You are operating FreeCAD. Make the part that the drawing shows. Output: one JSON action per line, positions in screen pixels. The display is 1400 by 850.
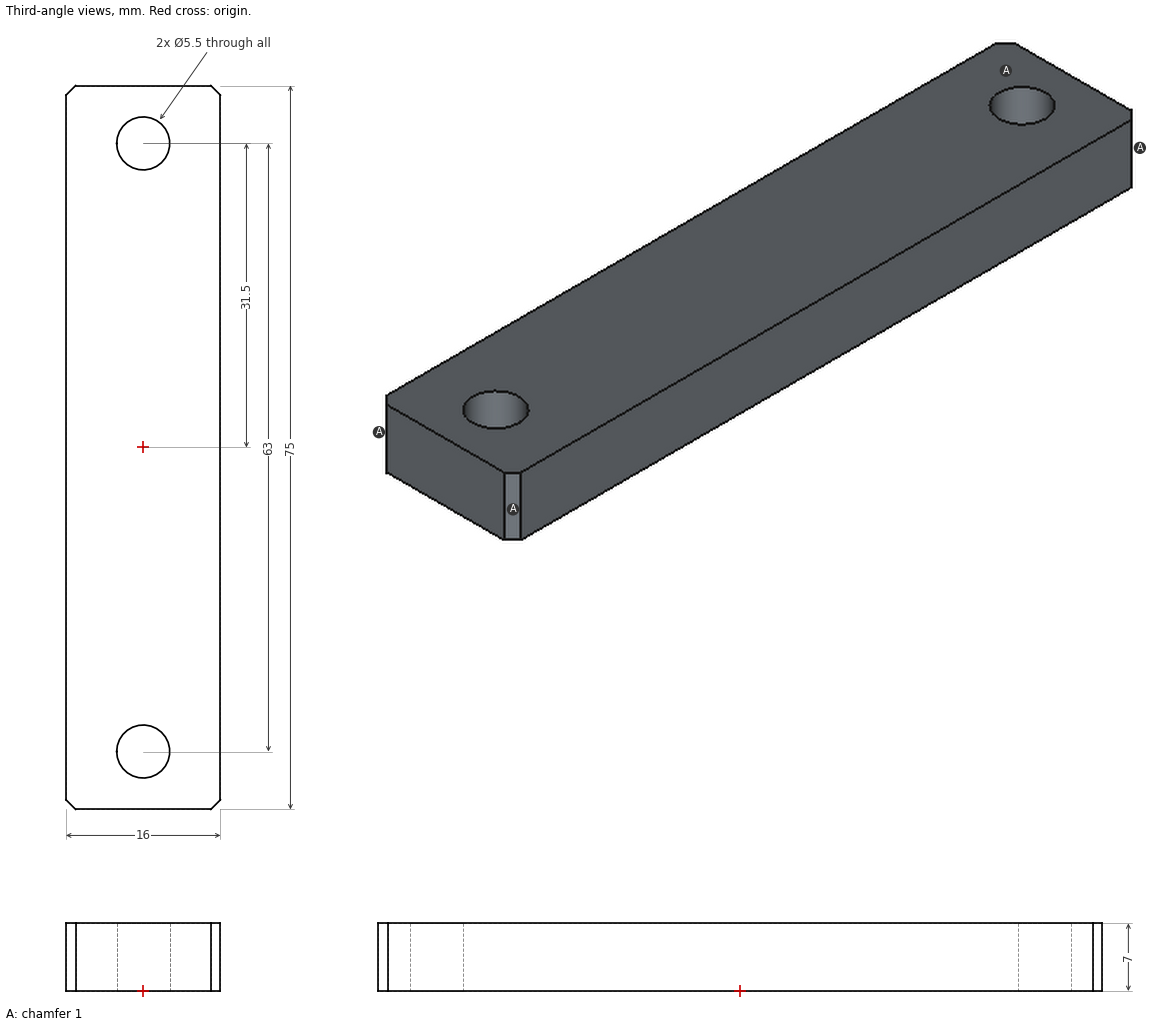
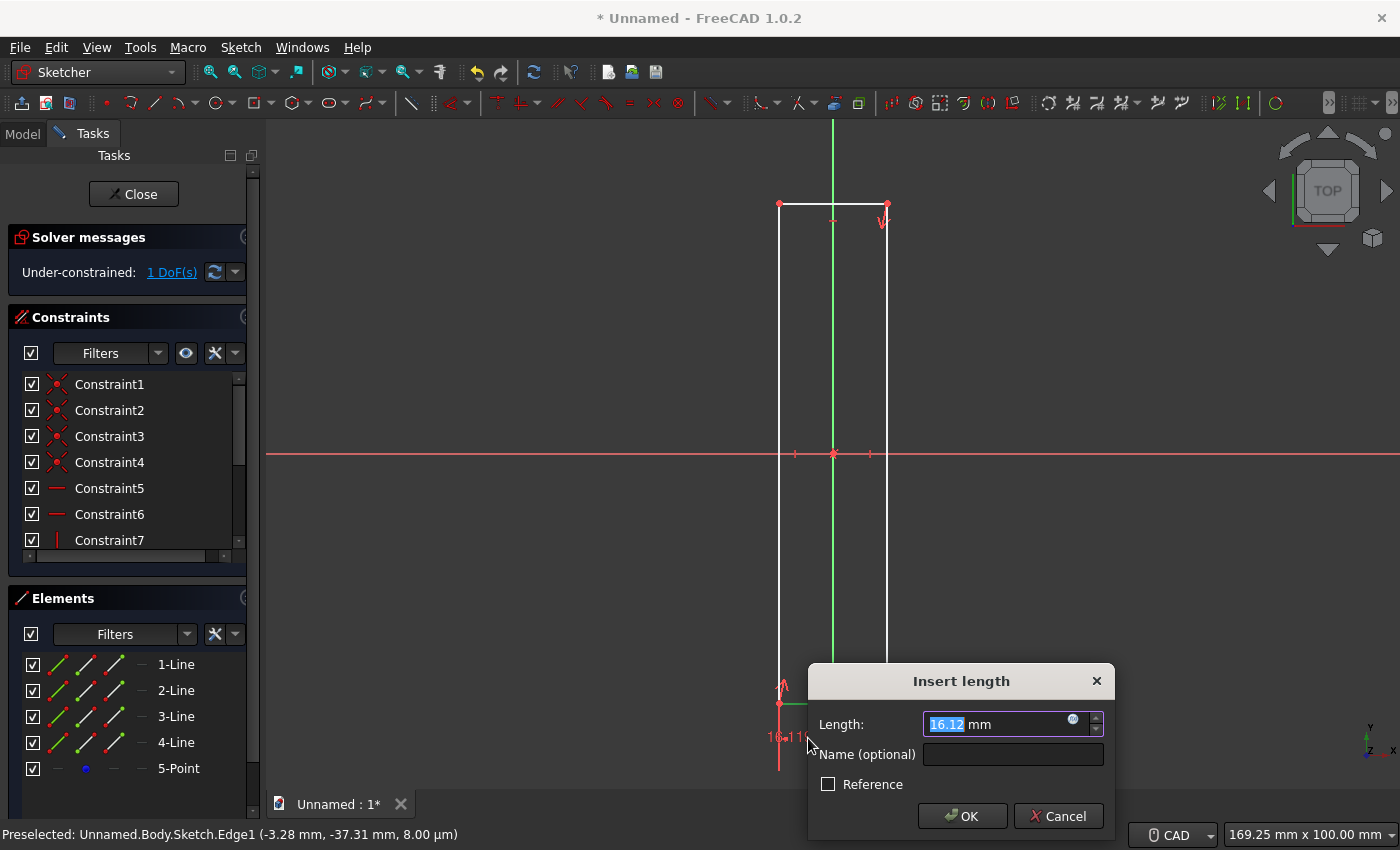
{"action": "type", "text": "16"}
{"action": "key", "text": "Return"}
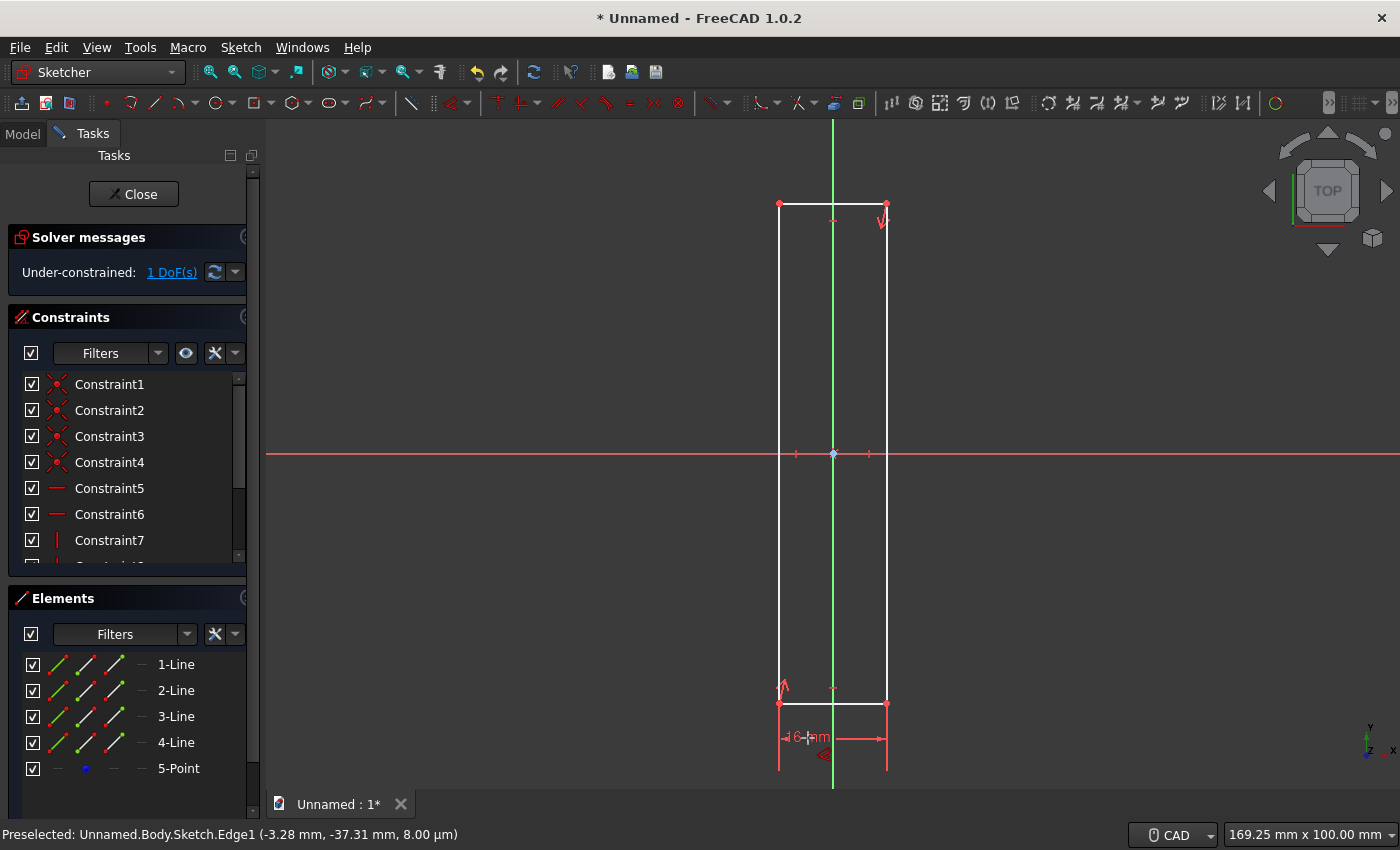
{"action": "left_click", "coordinate": [887, 554]}
{"action": "left_click", "coordinate": [921, 339]}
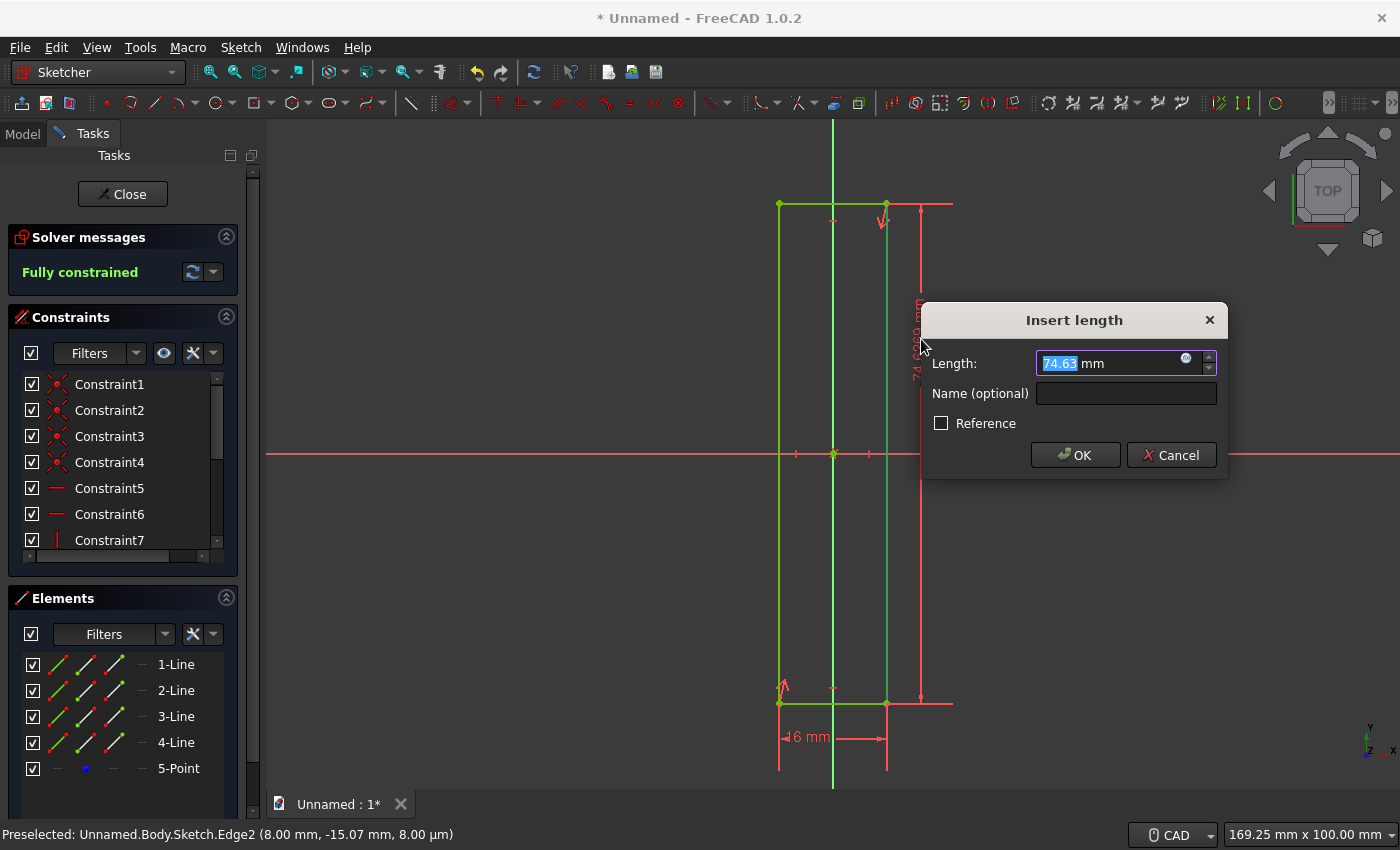
{"action": "type", "text": "75"}
{"action": "key", "text": "Return"}
{"action": "key", "text": "Escape"}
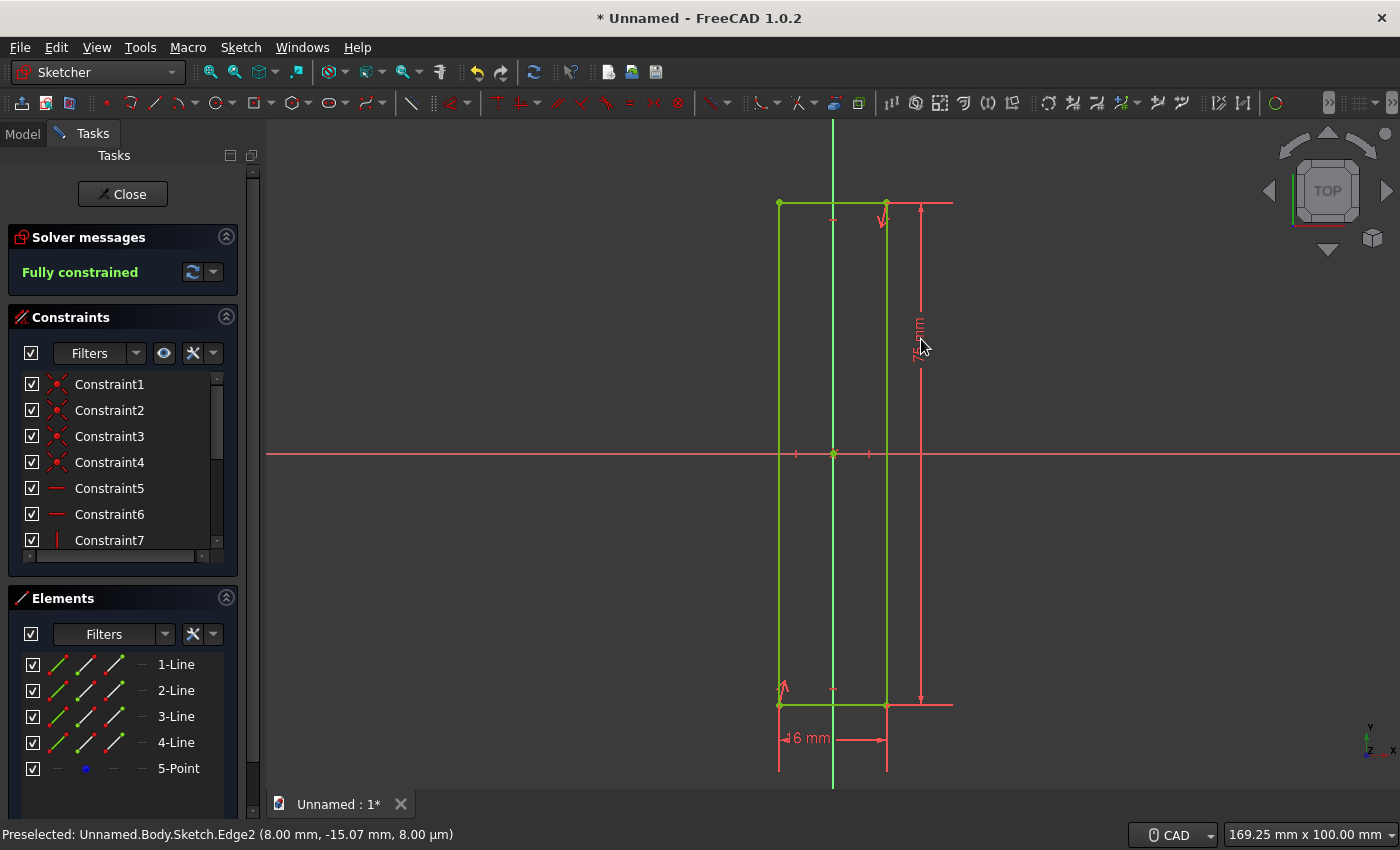
{"action": "left_click", "coordinate": [123, 194]}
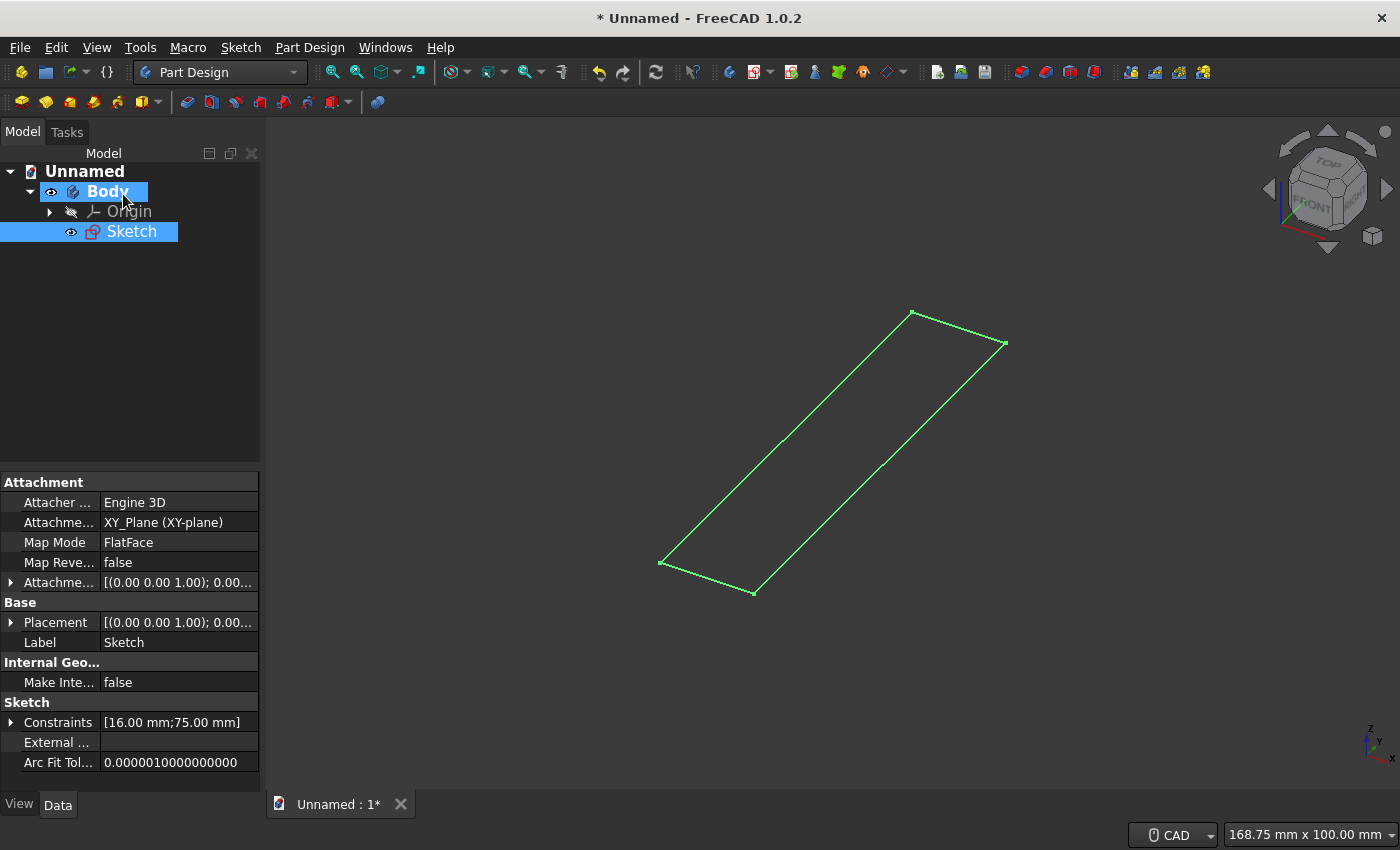
{"action": "left_click", "coordinate": [22, 102]}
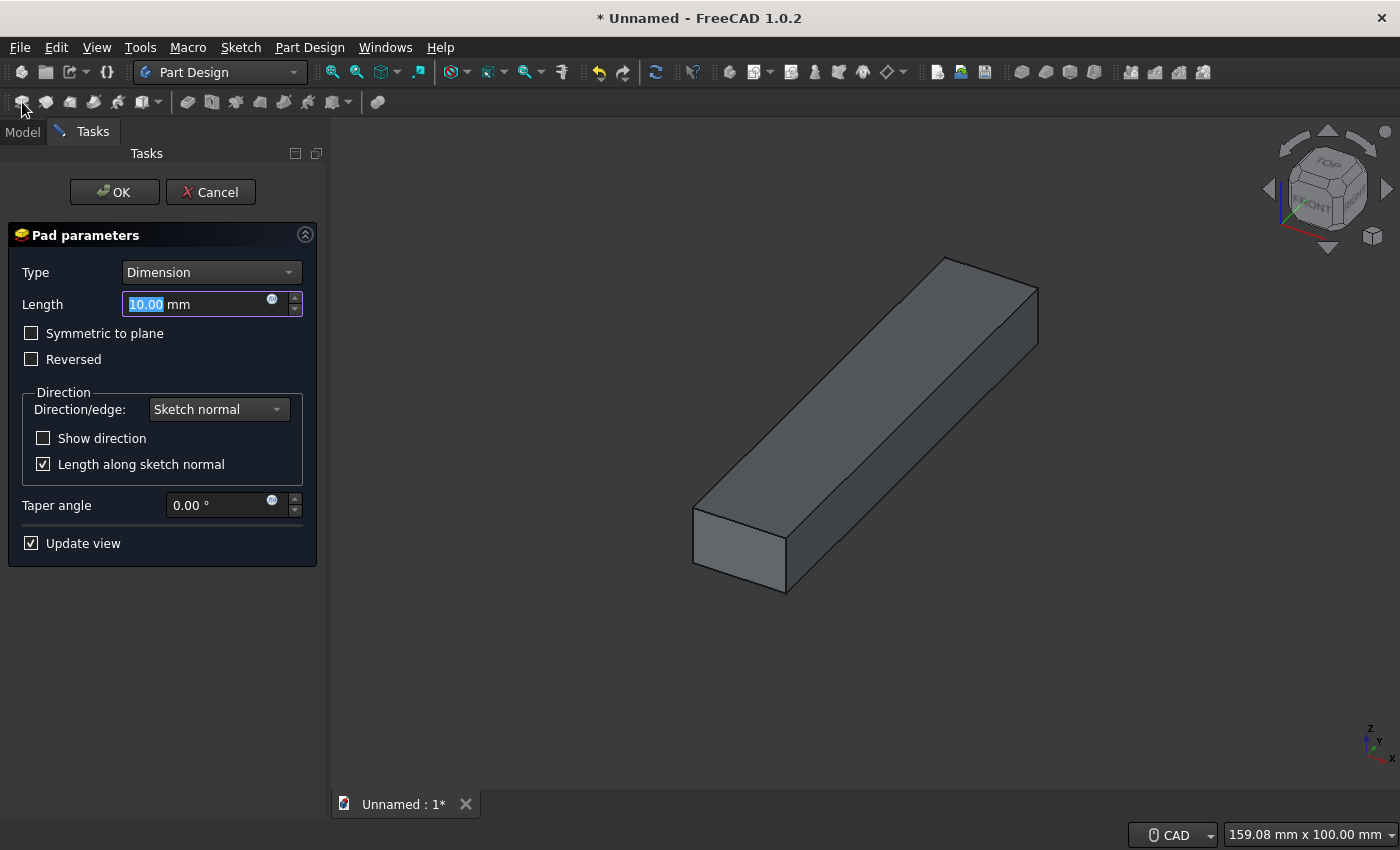
{"action": "type", "text": "7"}
{"action": "key", "text": "Tab"}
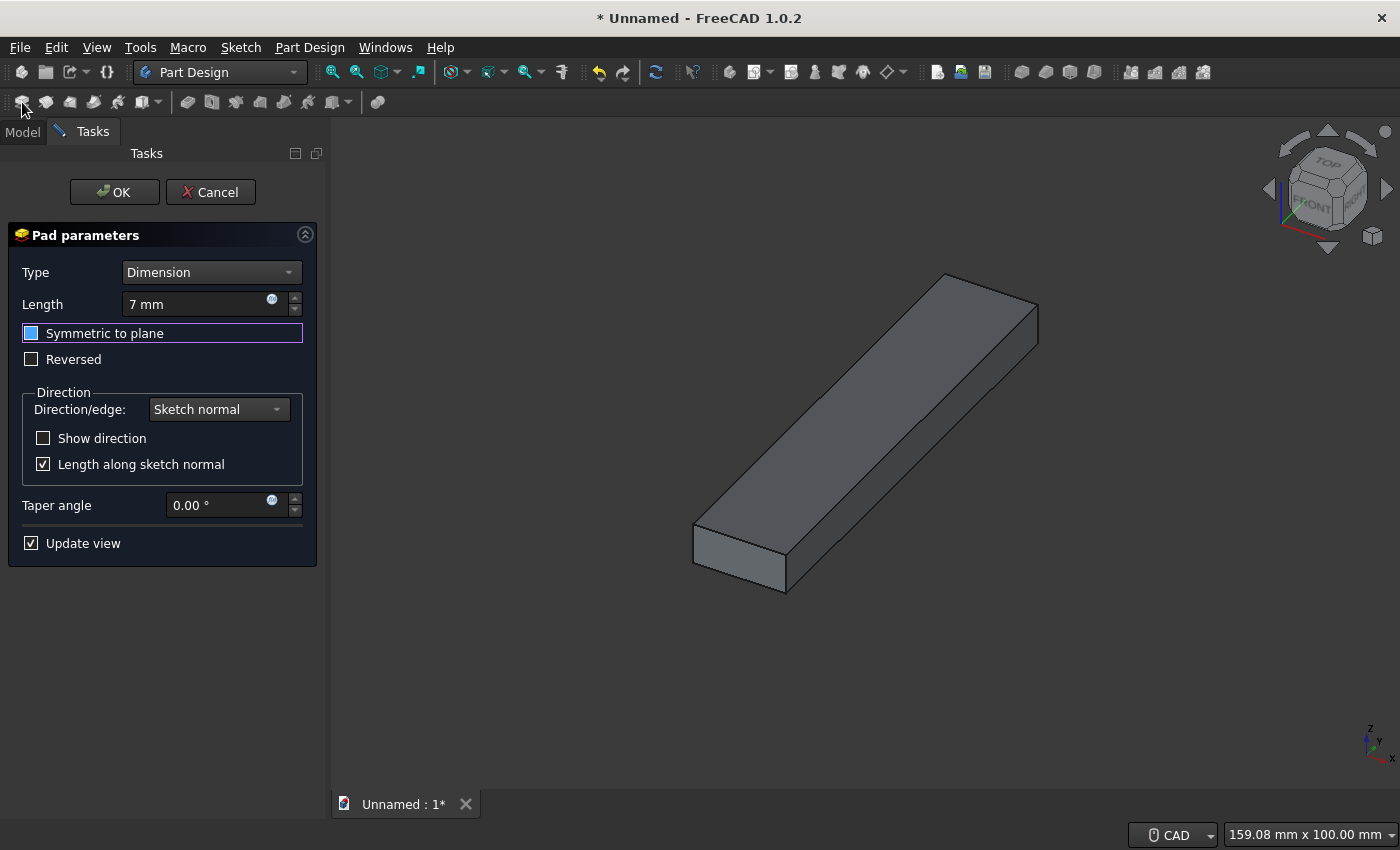
{"action": "left_click", "coordinate": [115, 192]}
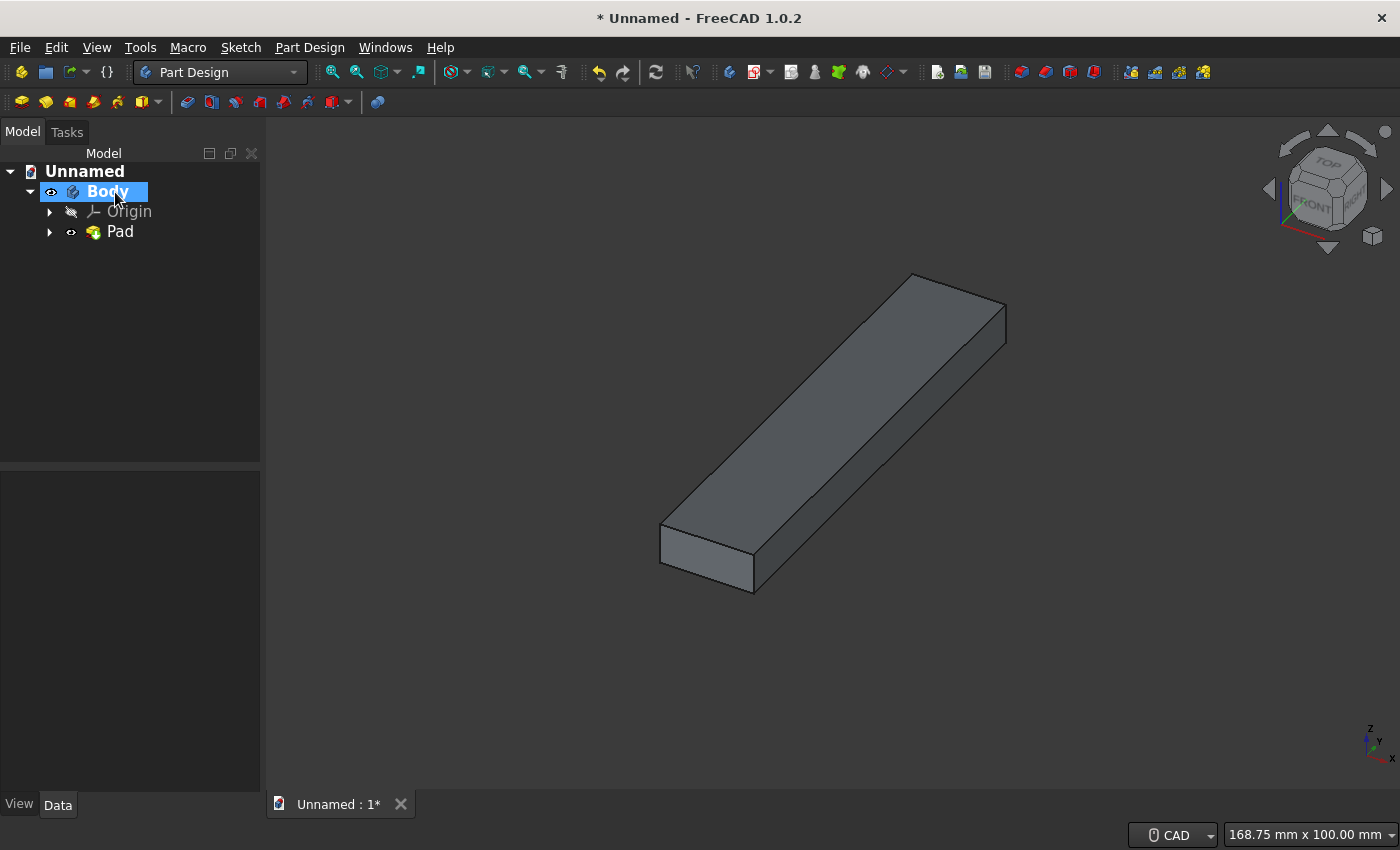
{"action": "left_click", "coordinate": [754, 573]}